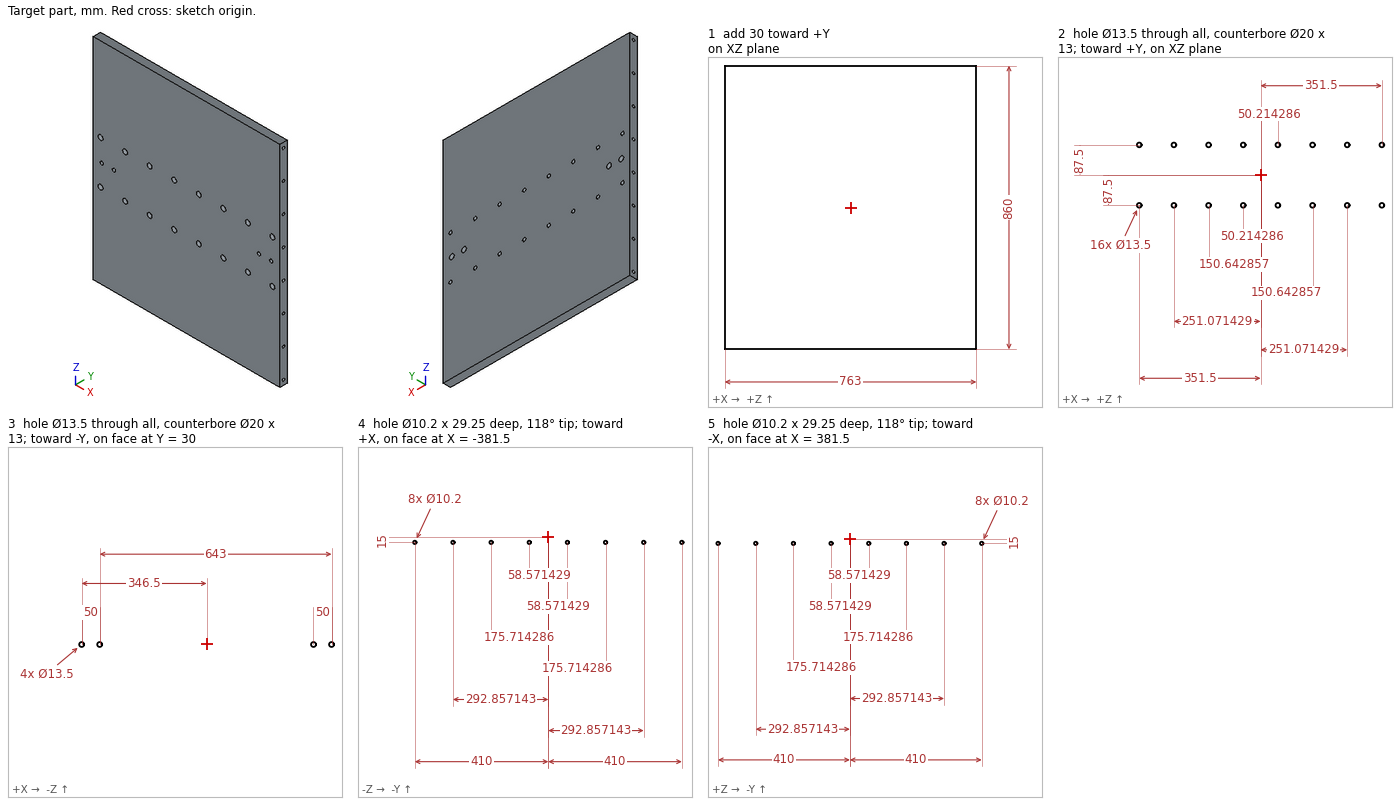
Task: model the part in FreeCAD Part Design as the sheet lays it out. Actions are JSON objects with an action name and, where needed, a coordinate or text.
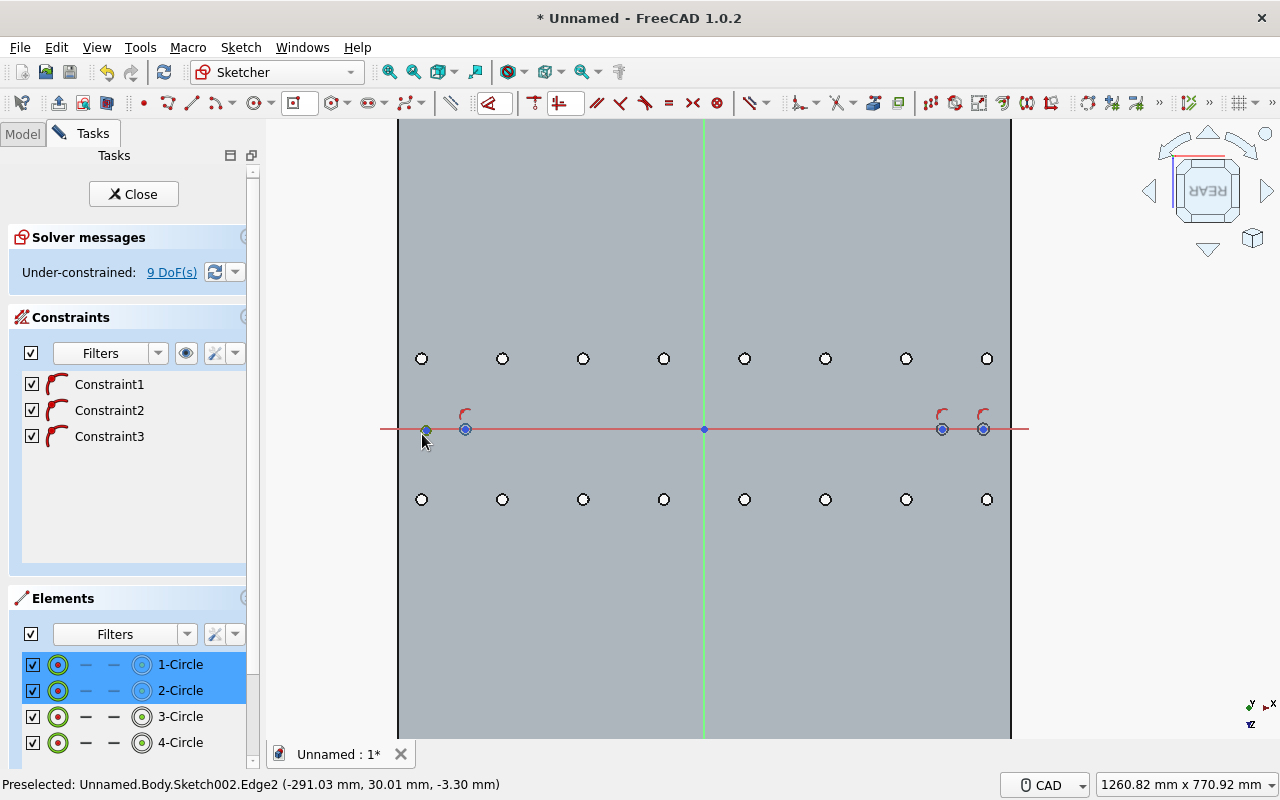
{"action": "scroll", "coordinate": [988, 425], "scroll_direction": "up", "scroll_amount": 7}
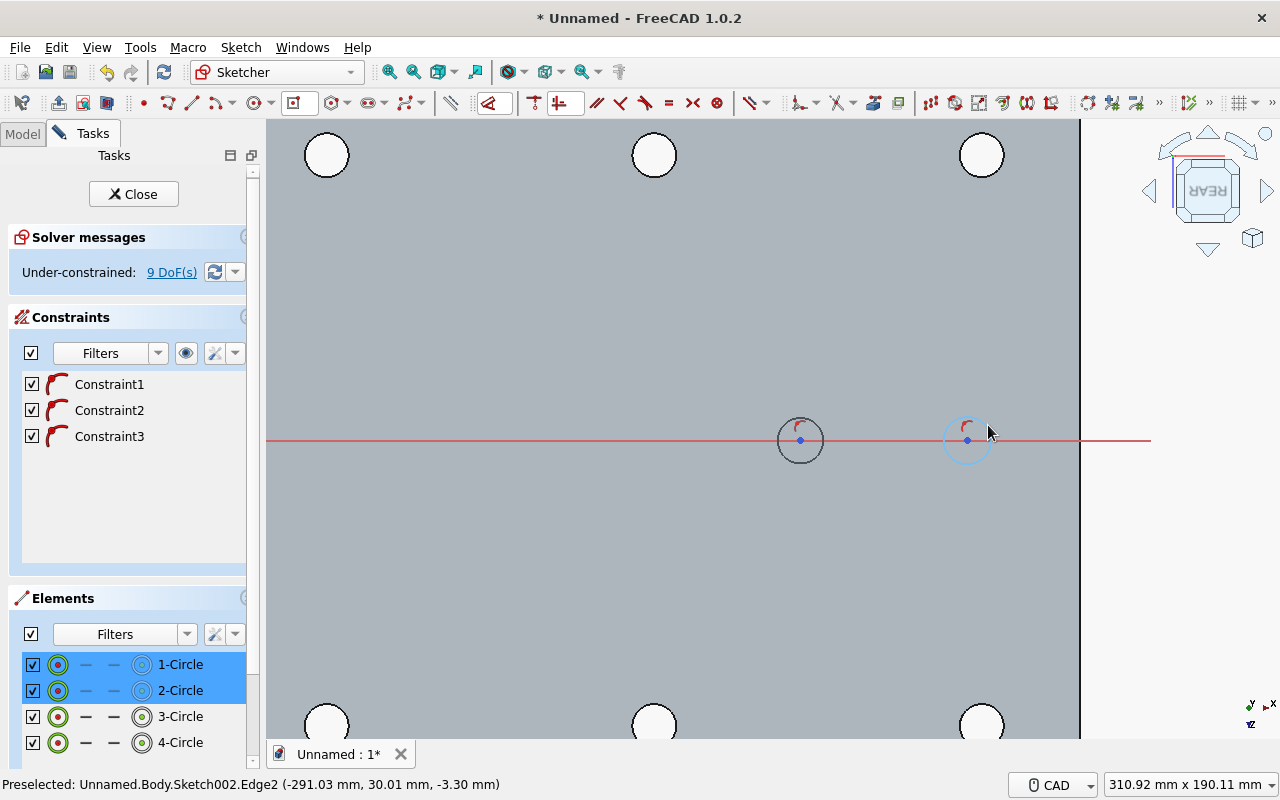
{"action": "left_click", "coordinate": [984, 424]}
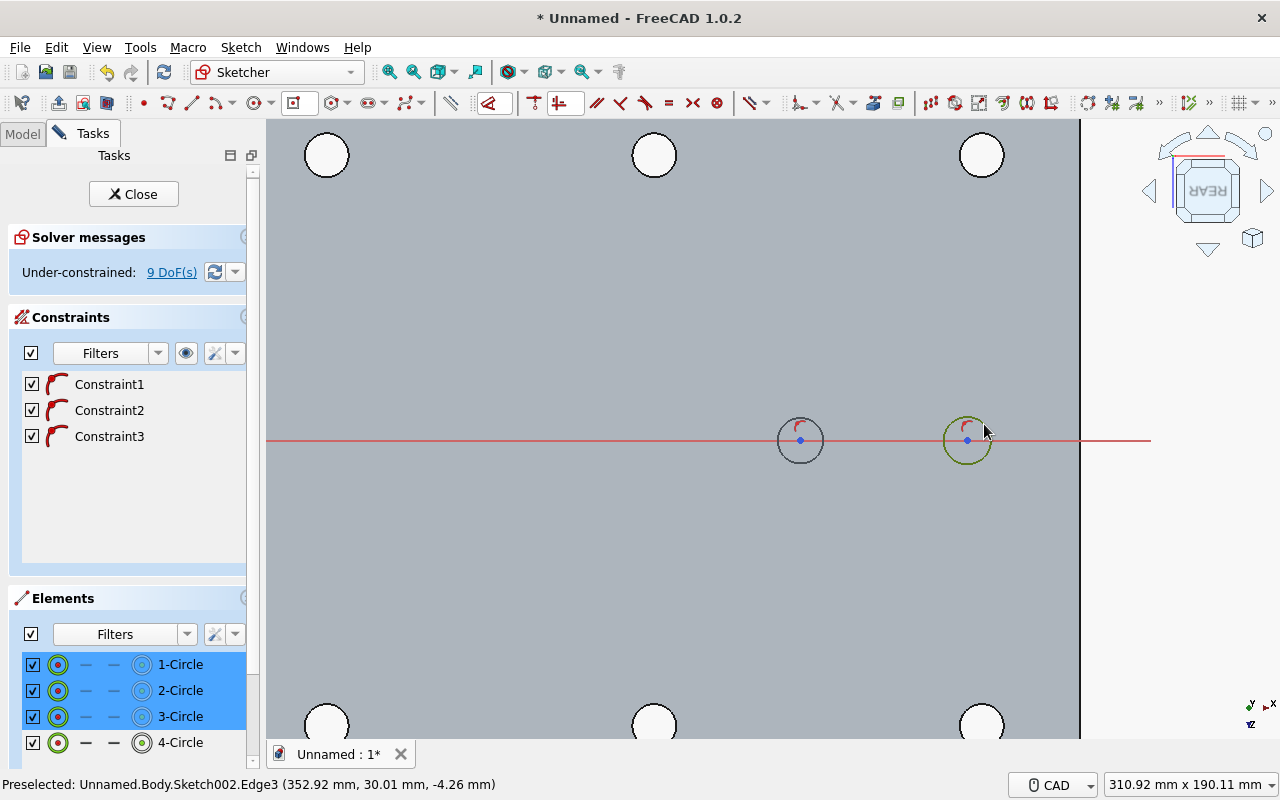
{"action": "left_click", "coordinate": [817, 425]}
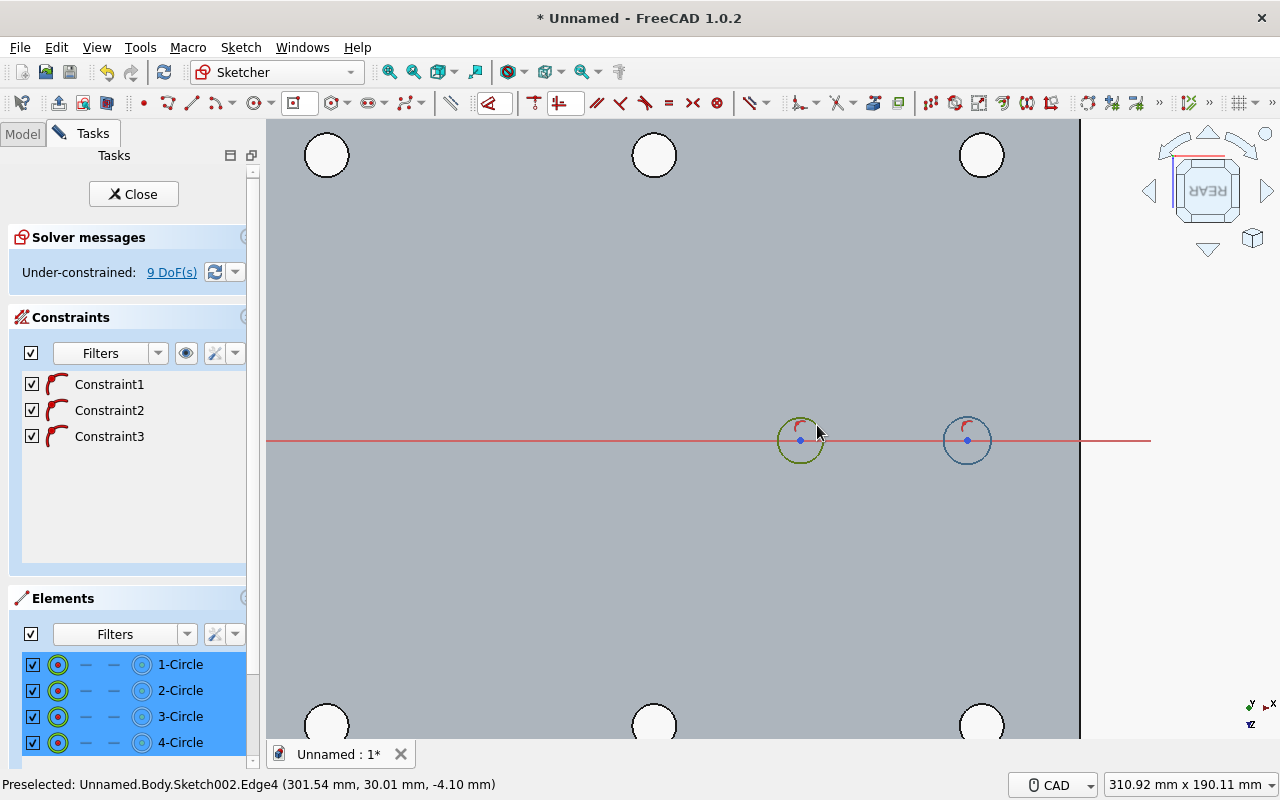
{"action": "left_click", "coordinate": [670, 104]}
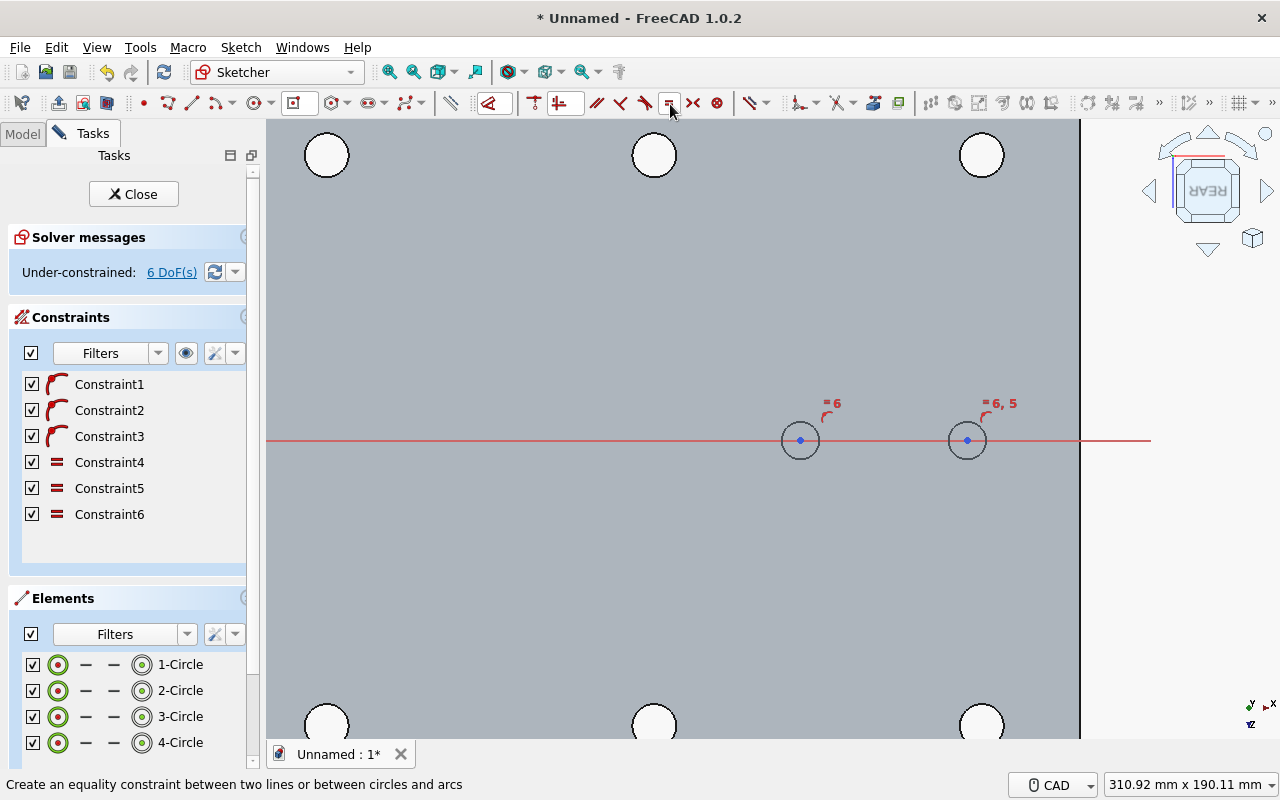
{"action": "scroll", "coordinate": [989, 425], "scroll_direction": "down", "scroll_amount": 7}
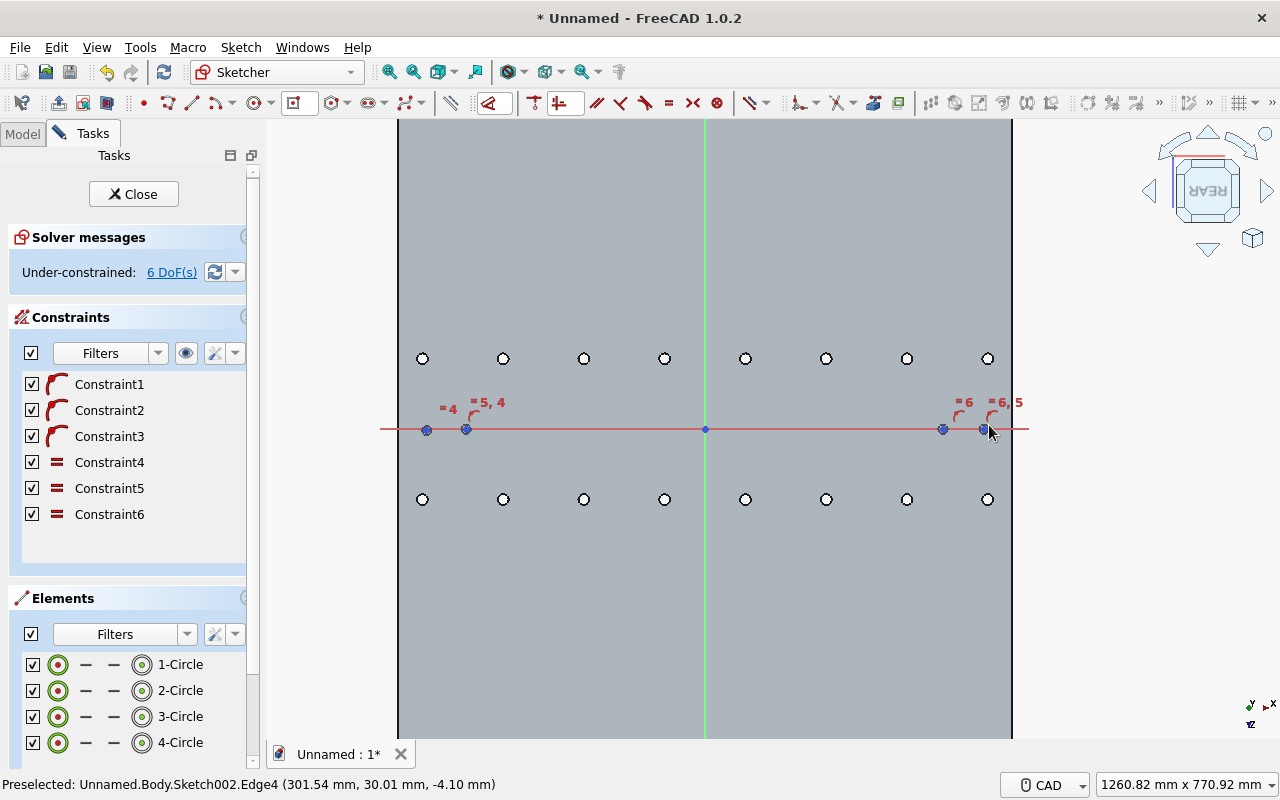
{"action": "left_click", "coordinate": [427, 431]}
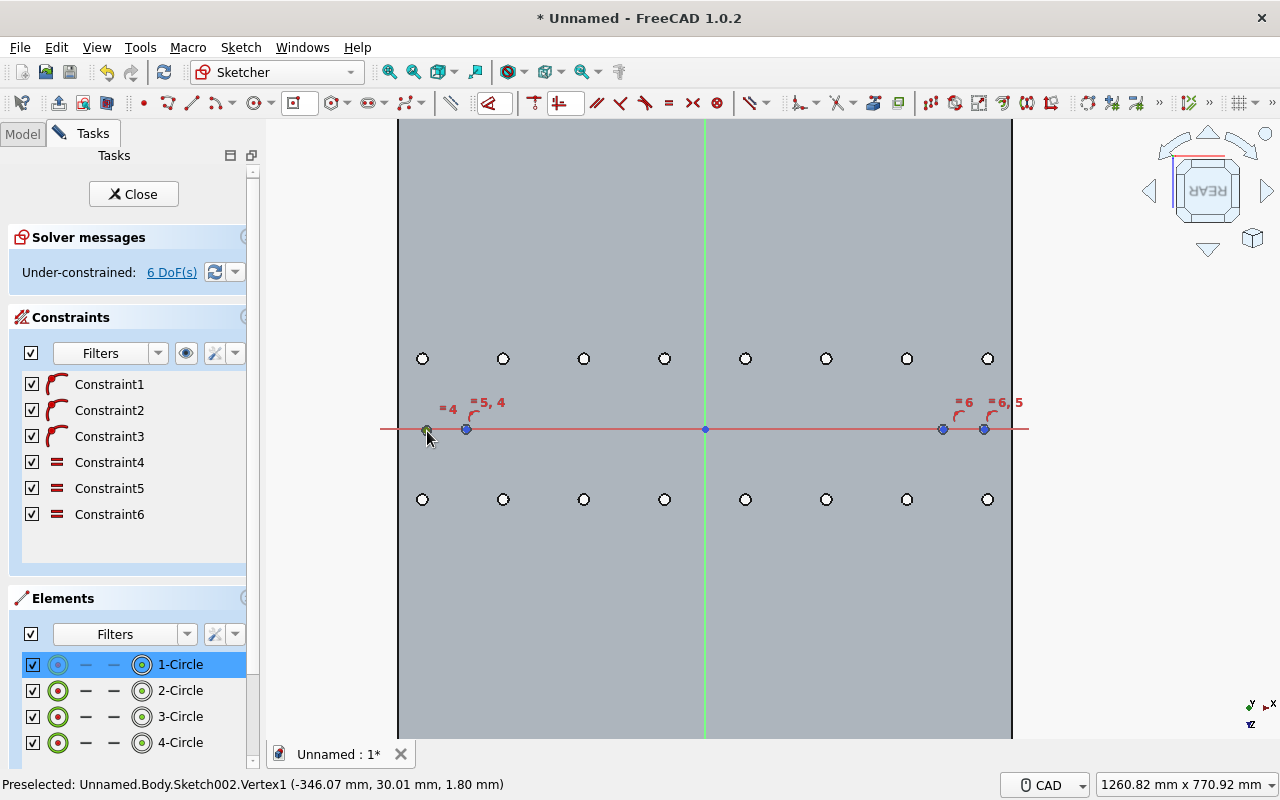
{"action": "left_click", "coordinate": [529, 429]}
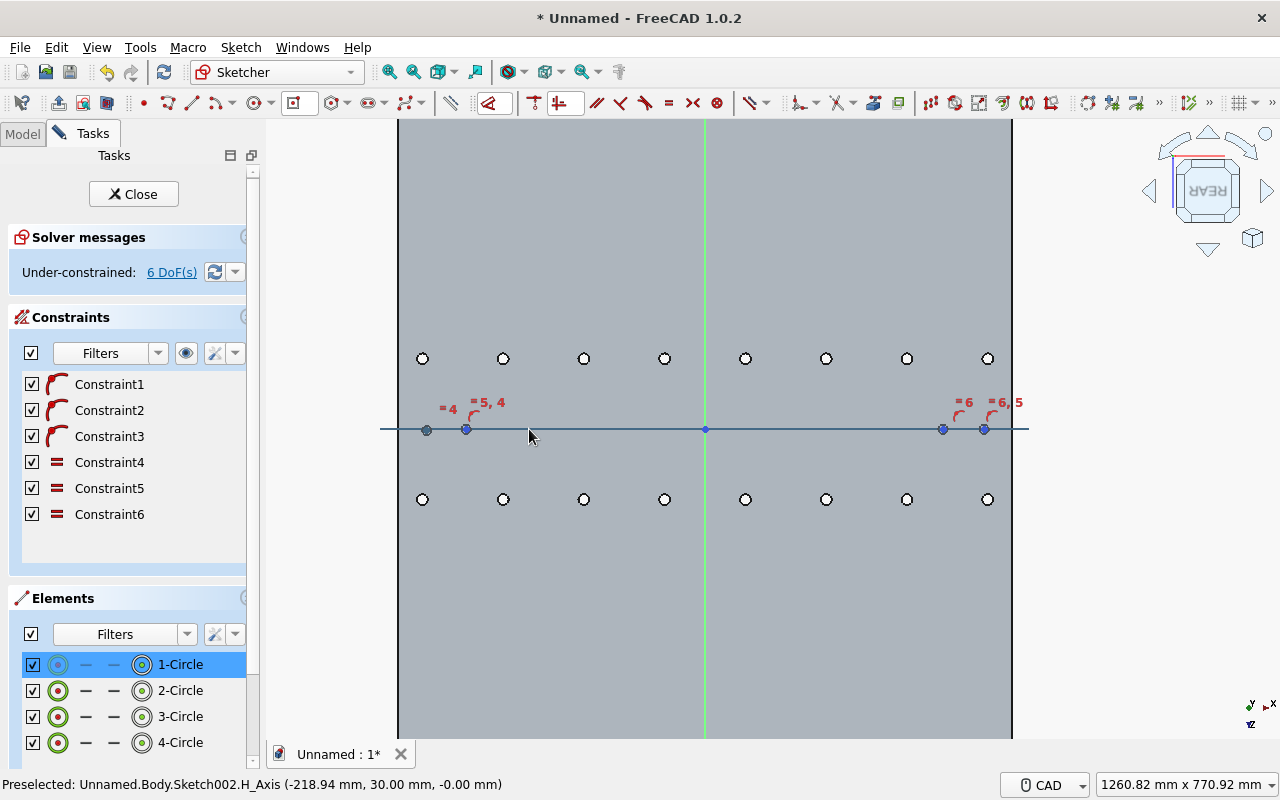
{"action": "left_click", "coordinate": [534, 104]}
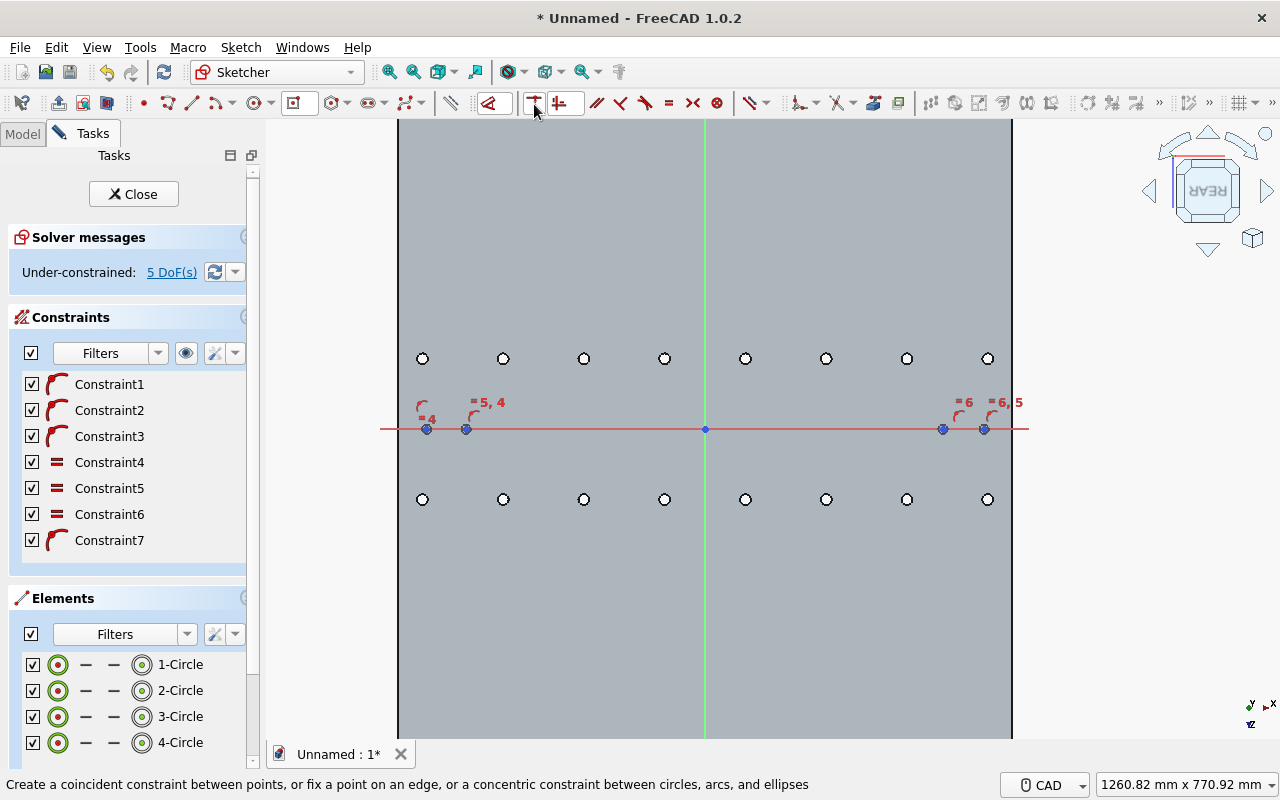
{"action": "scroll", "coordinate": [430, 426], "scroll_direction": "up", "scroll_amount": 7}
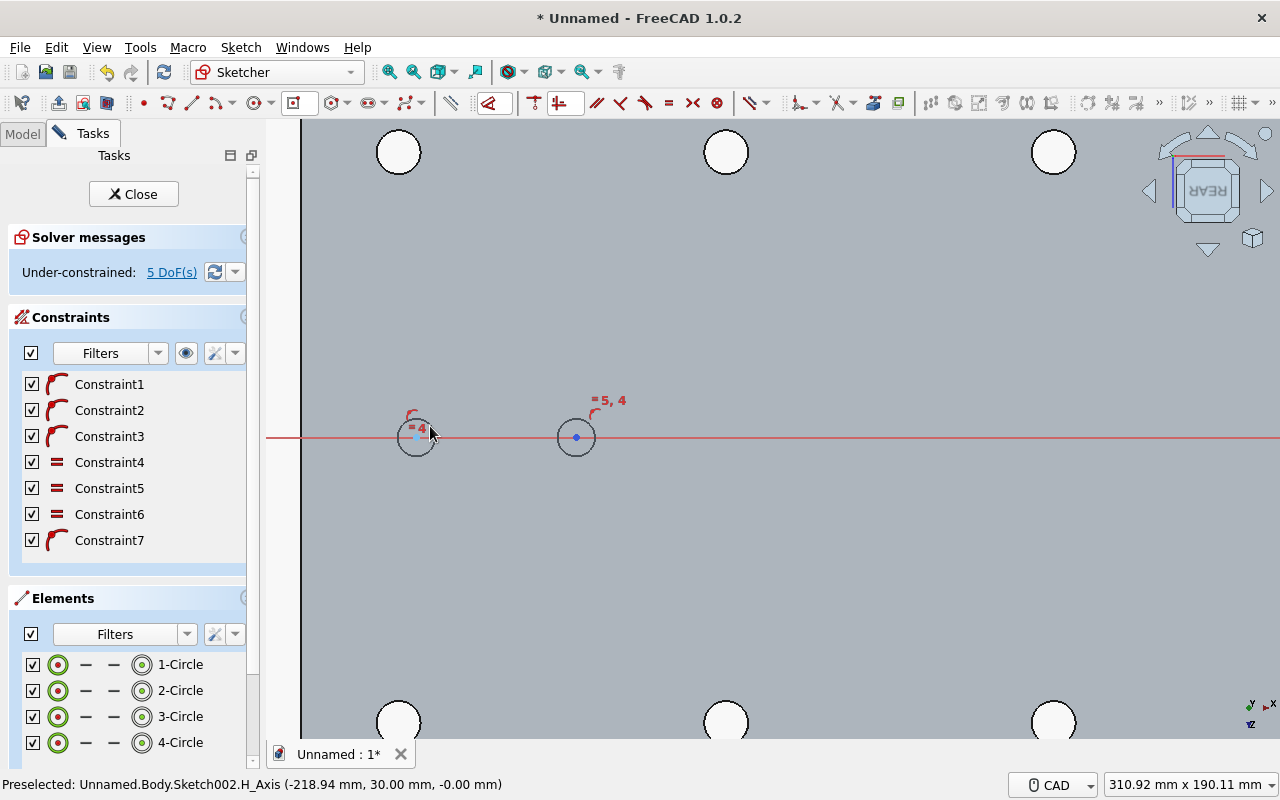
{"action": "left_click", "coordinate": [430, 424]}